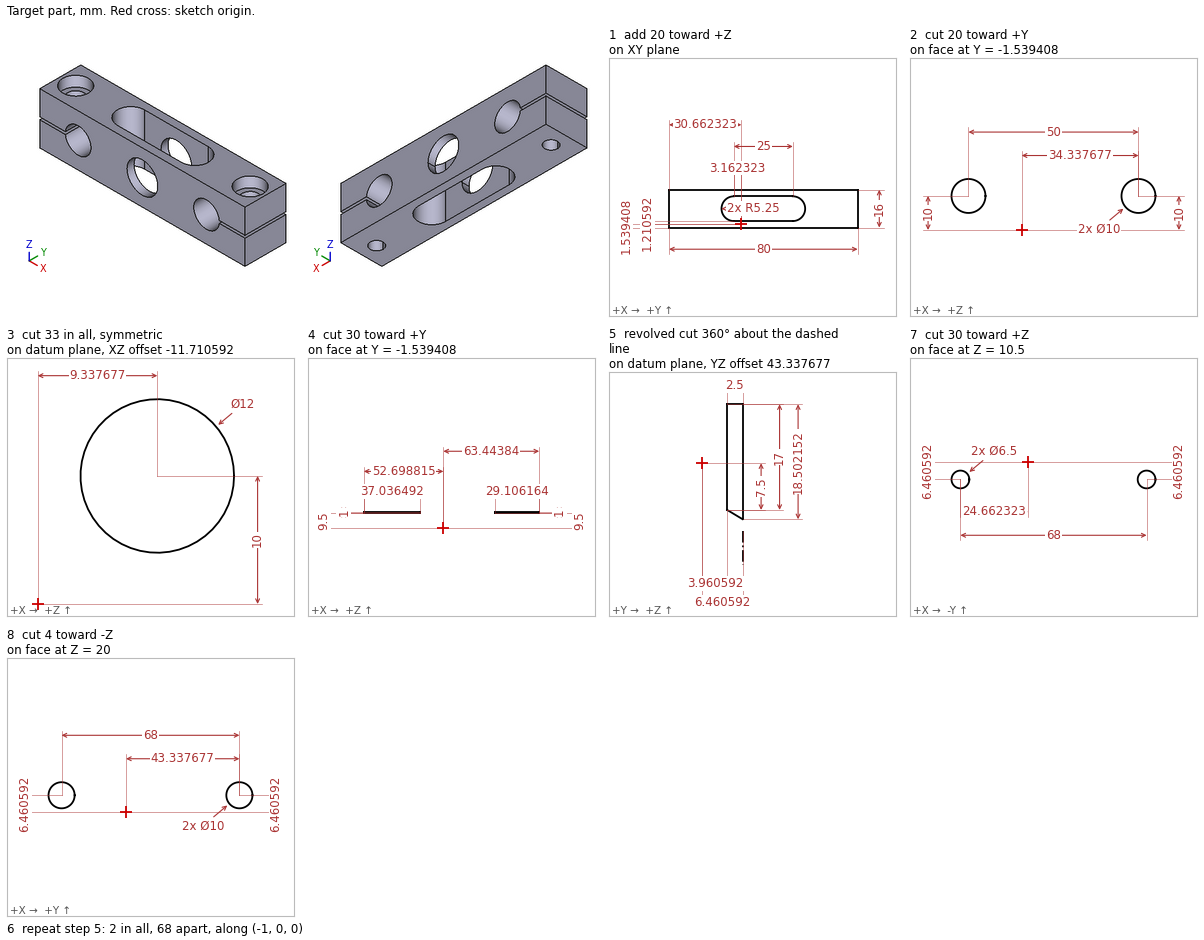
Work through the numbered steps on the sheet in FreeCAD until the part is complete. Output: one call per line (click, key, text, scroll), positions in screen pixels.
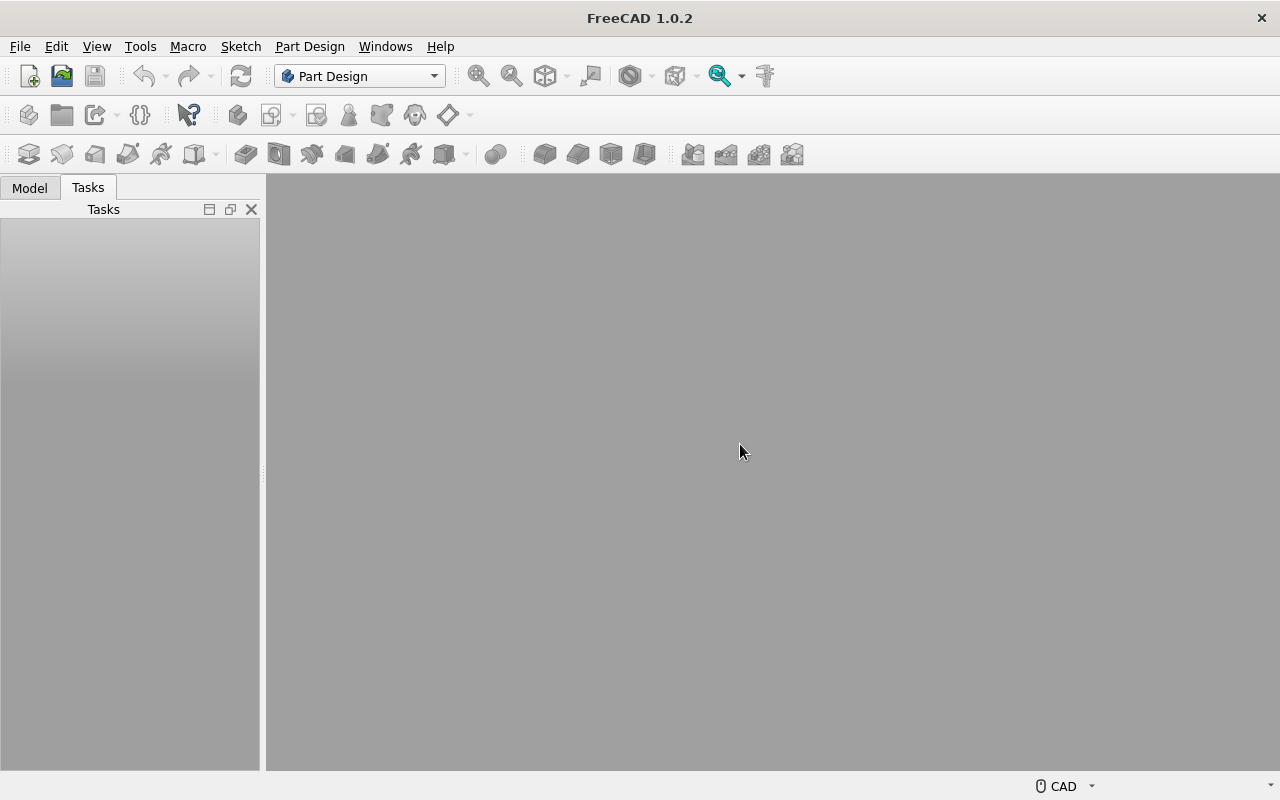
click(29, 76)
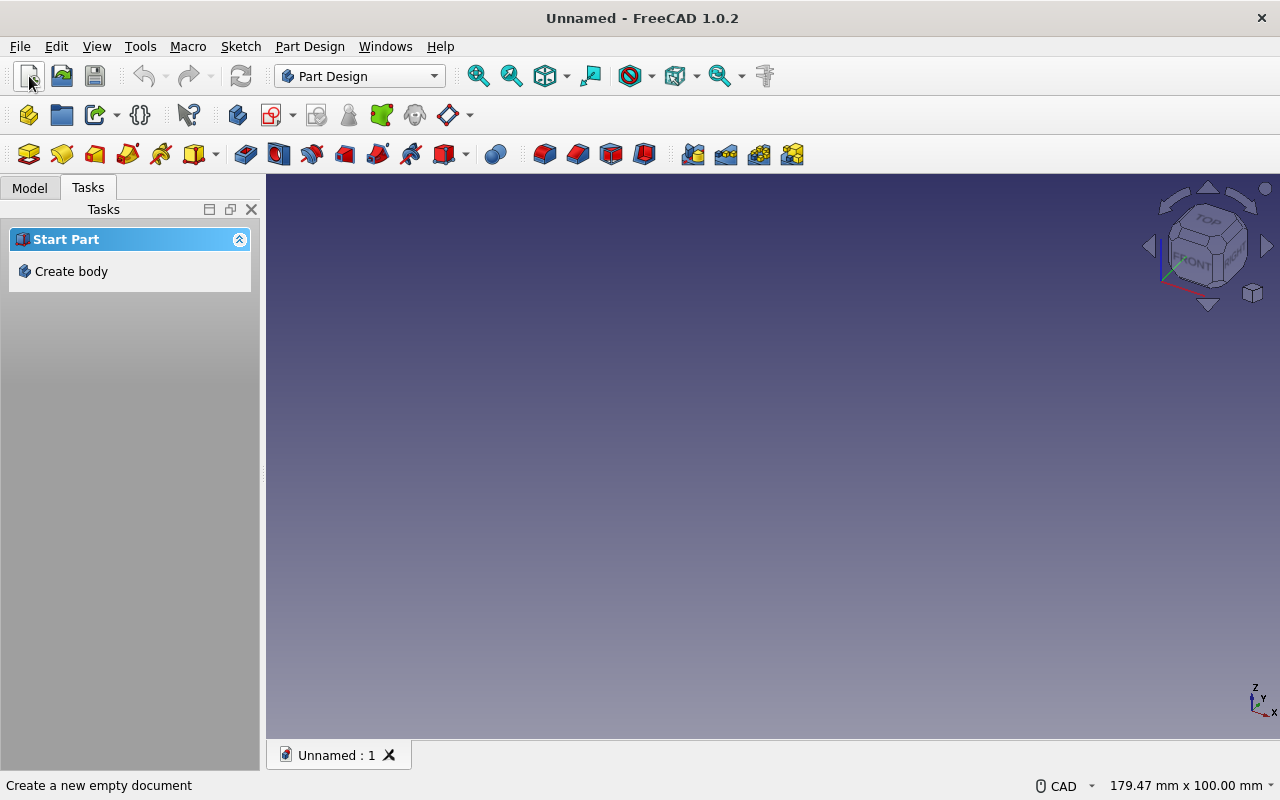
click(270, 116)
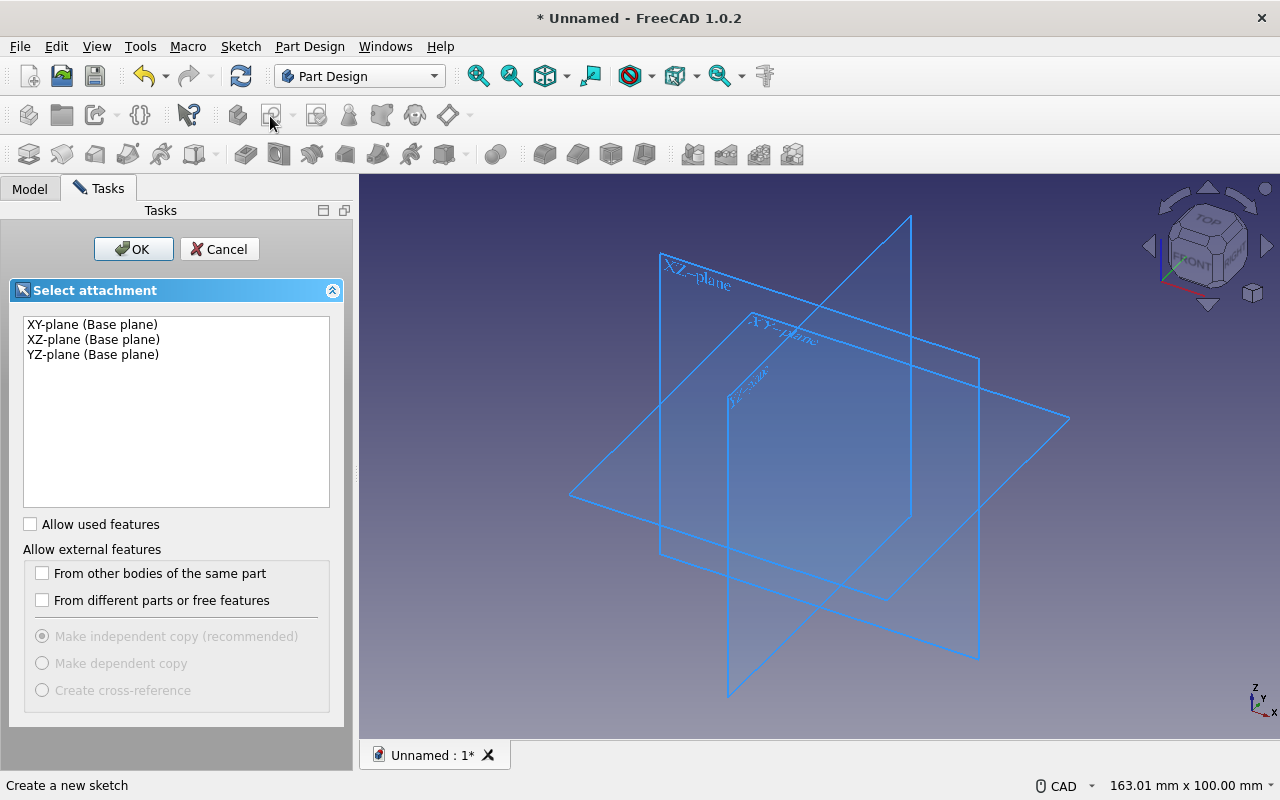
click(84, 324)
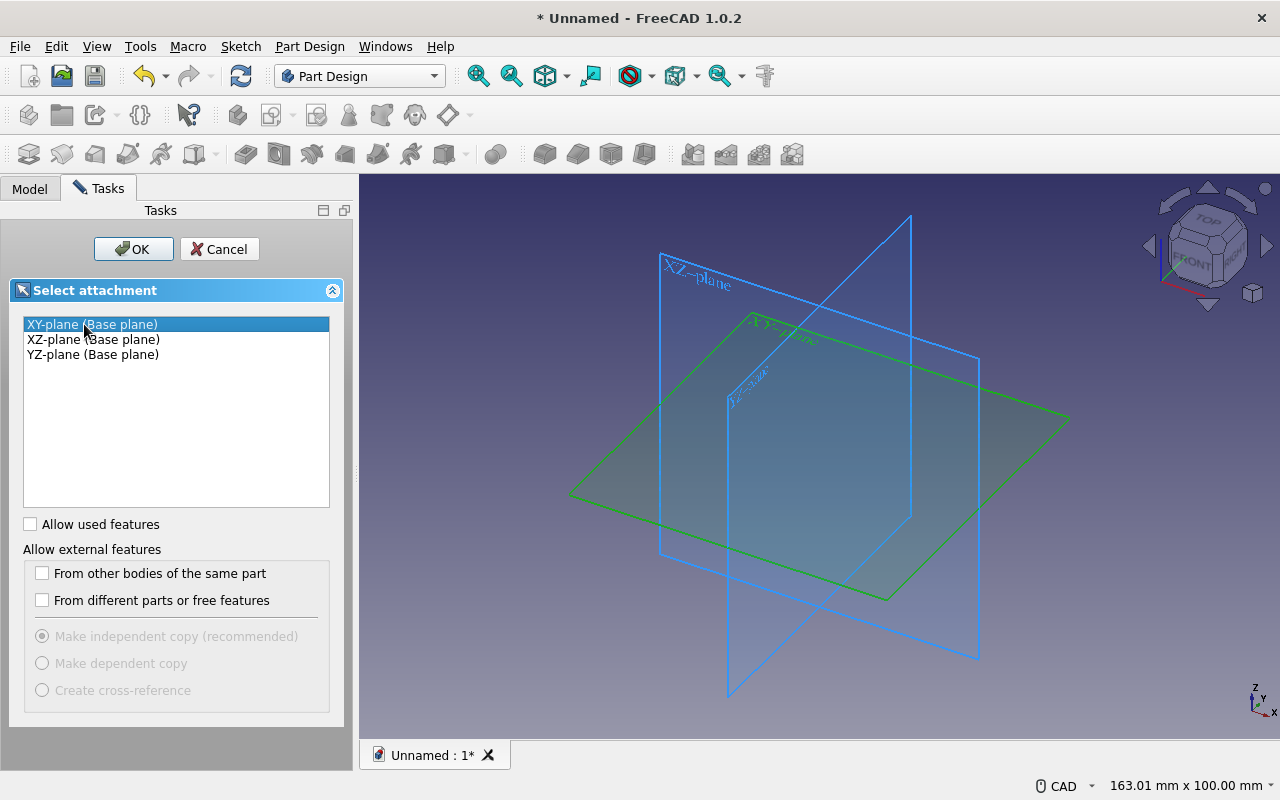
click(134, 249)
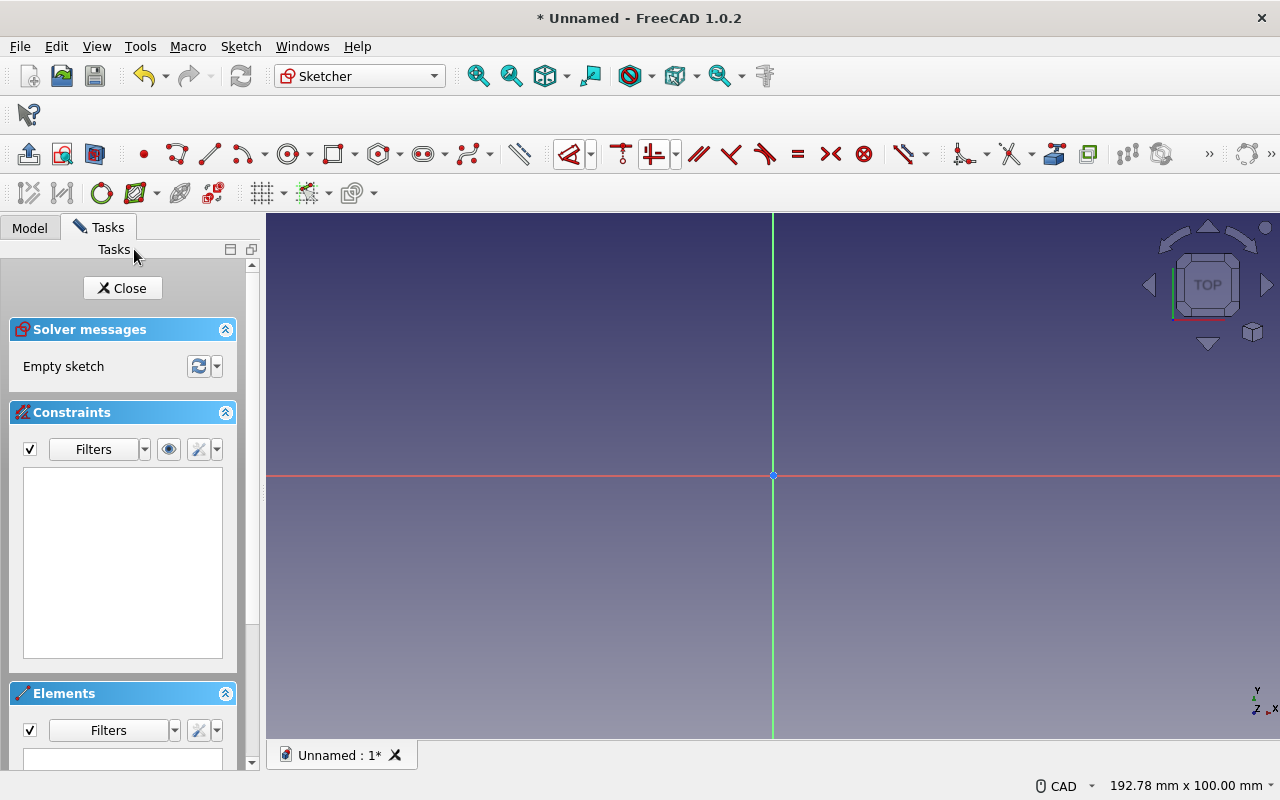
scroll(1061, 373, up, 2)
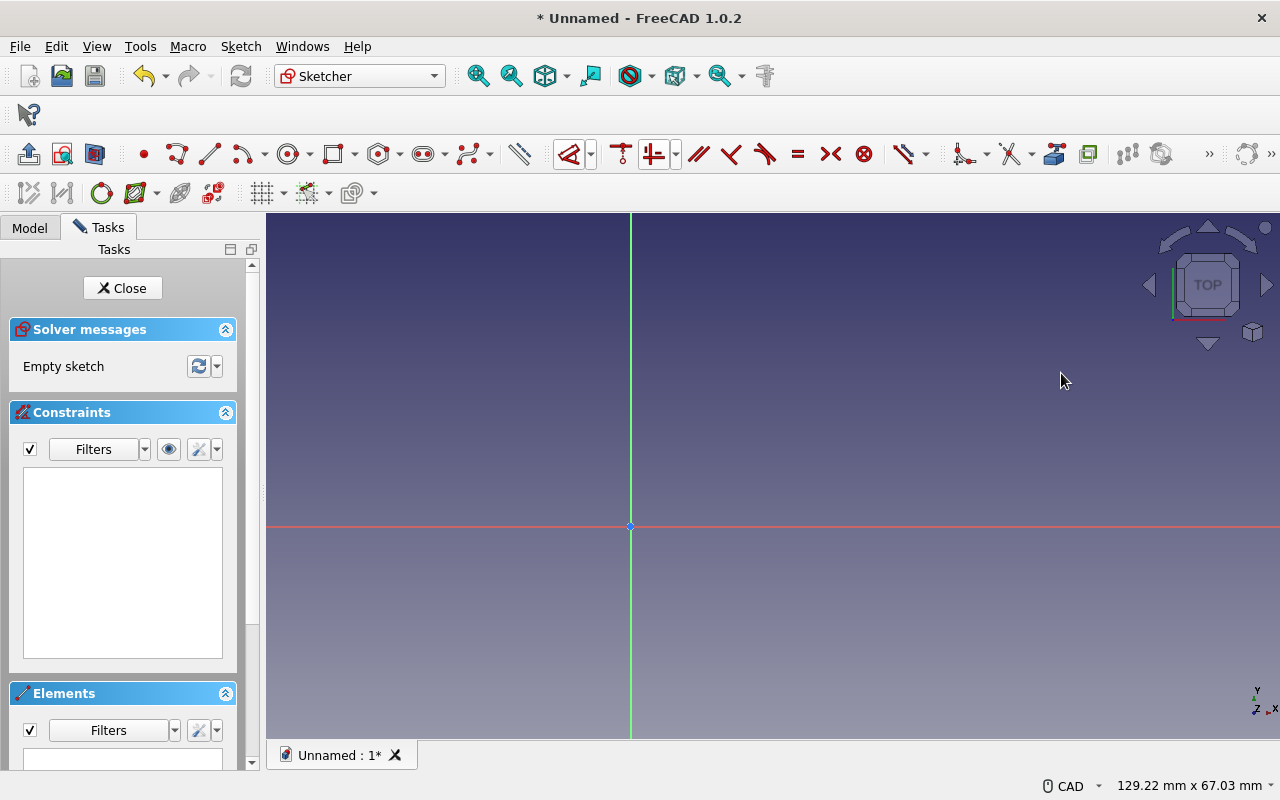
click(332, 154)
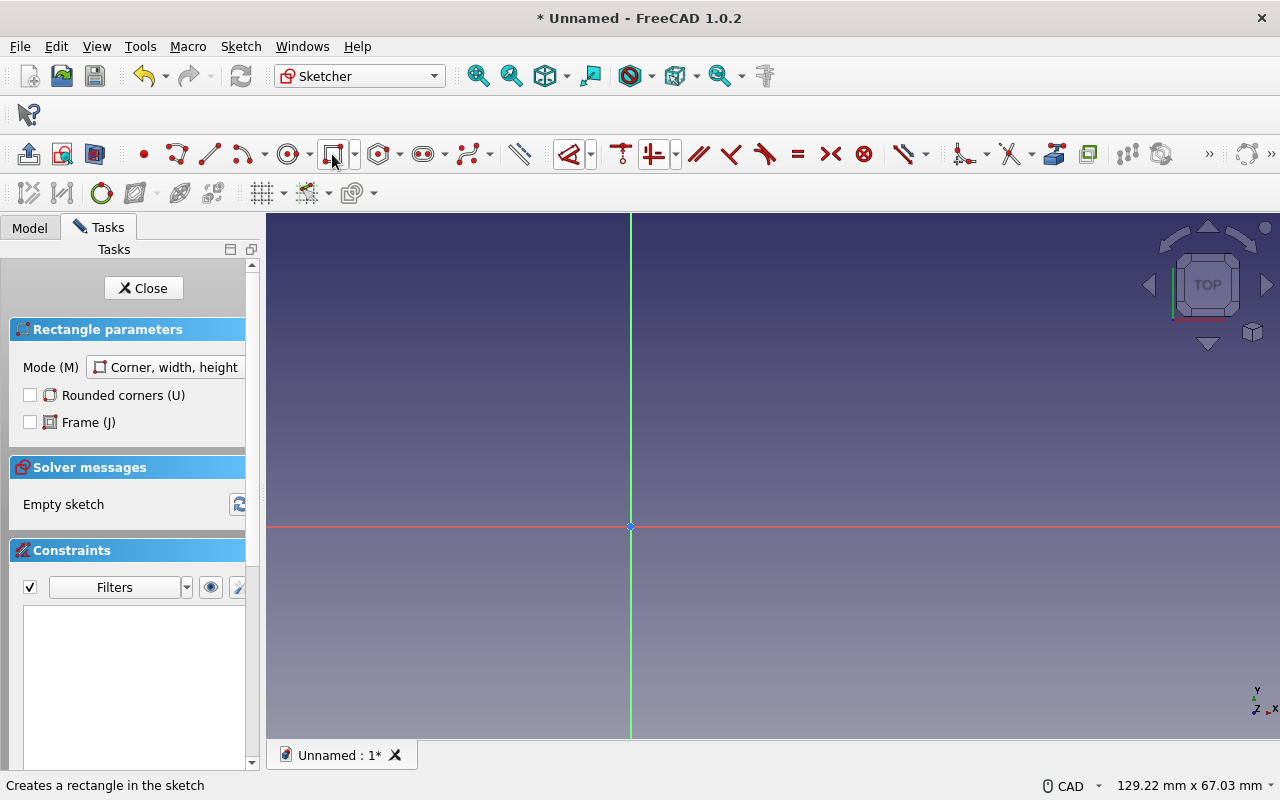
click(390, 413)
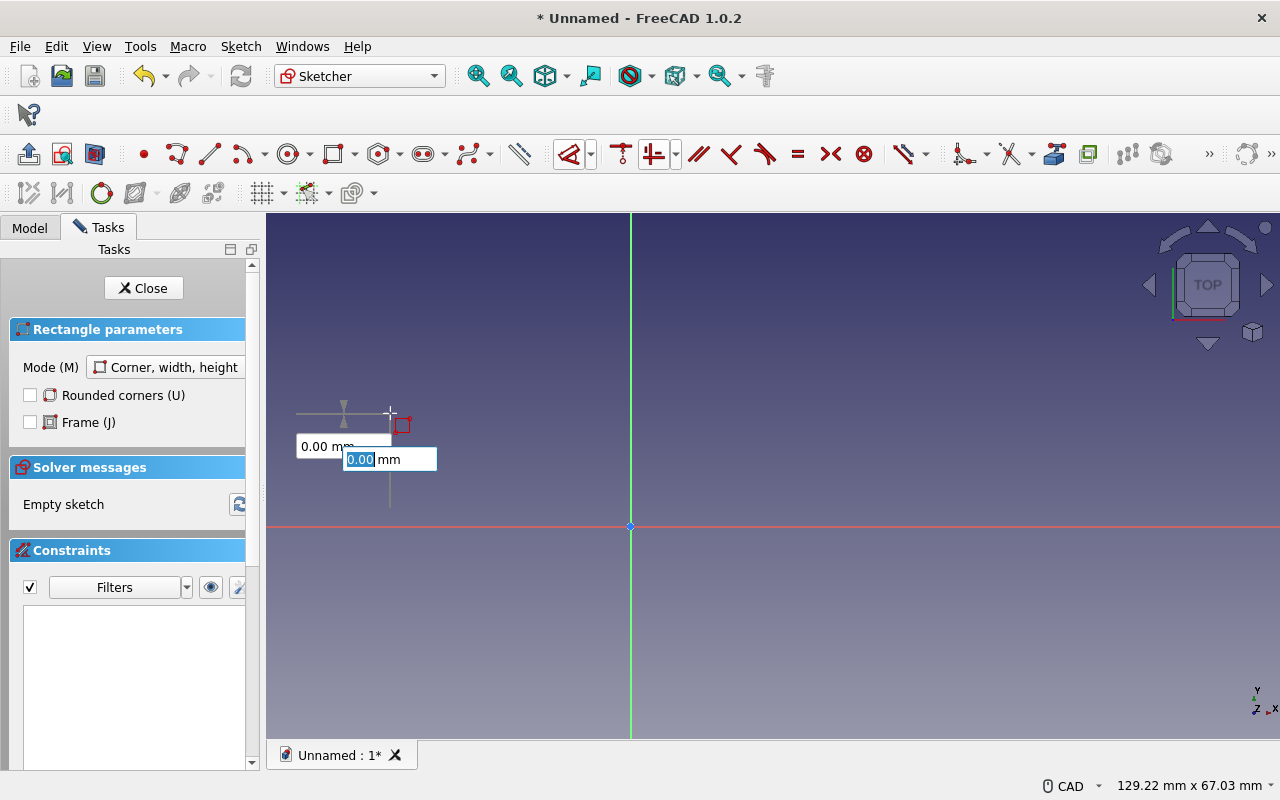
scroll(1018, 539, up, 2)
move(1018, 538)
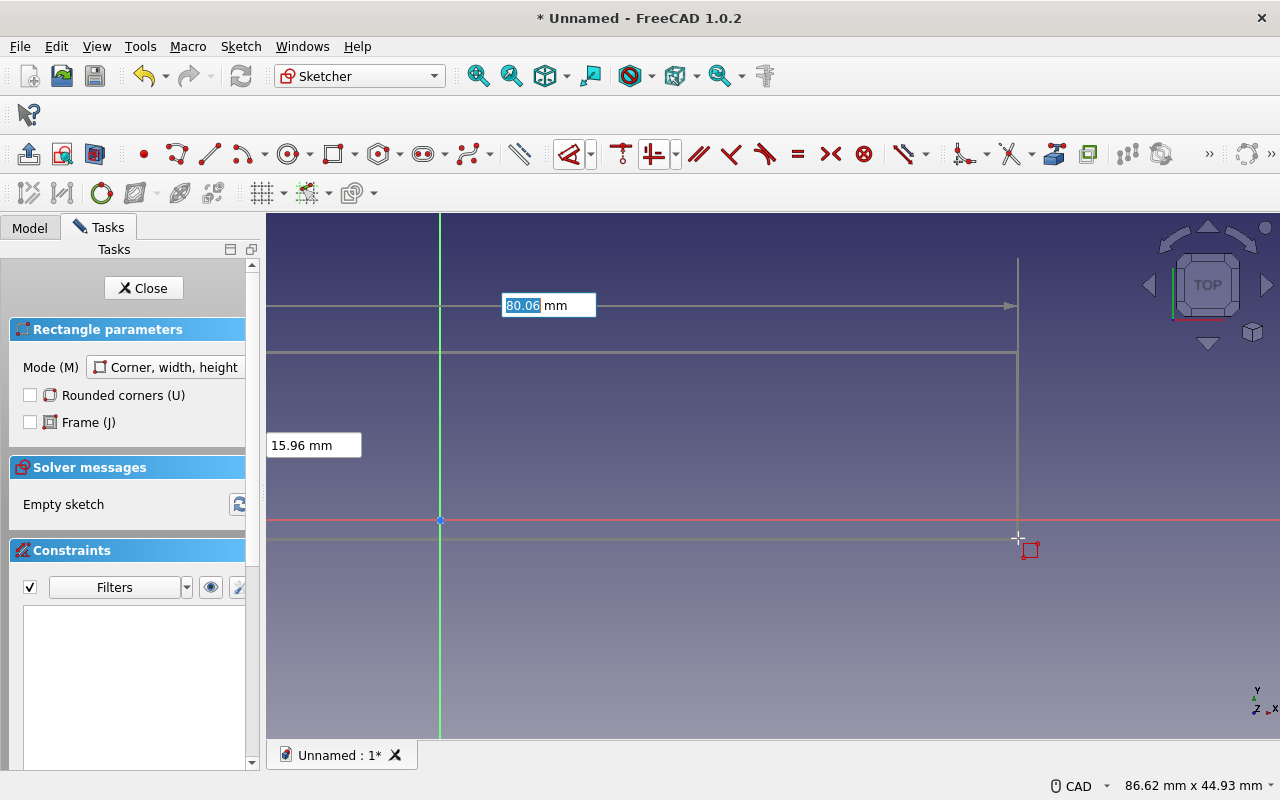
text(80)
key(Tab)
text(16)
key(Return)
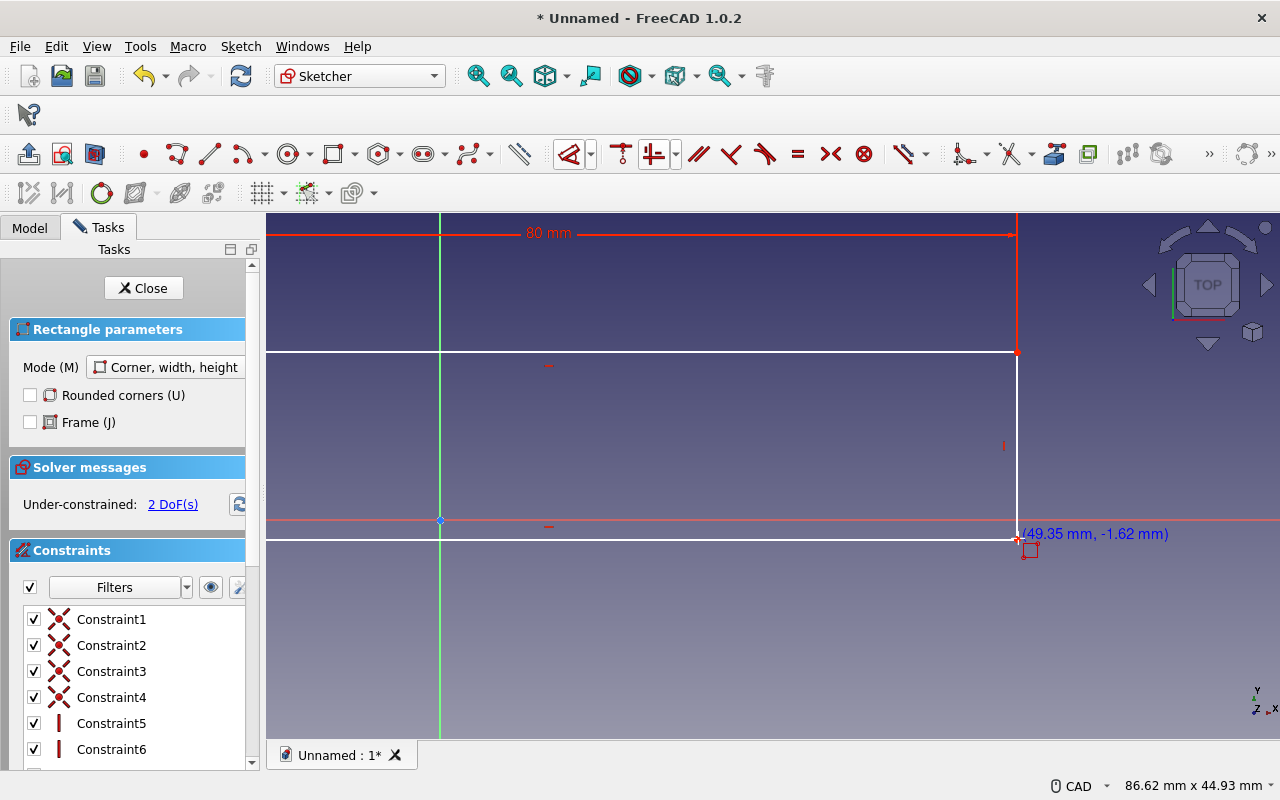
key(g)
key(s)